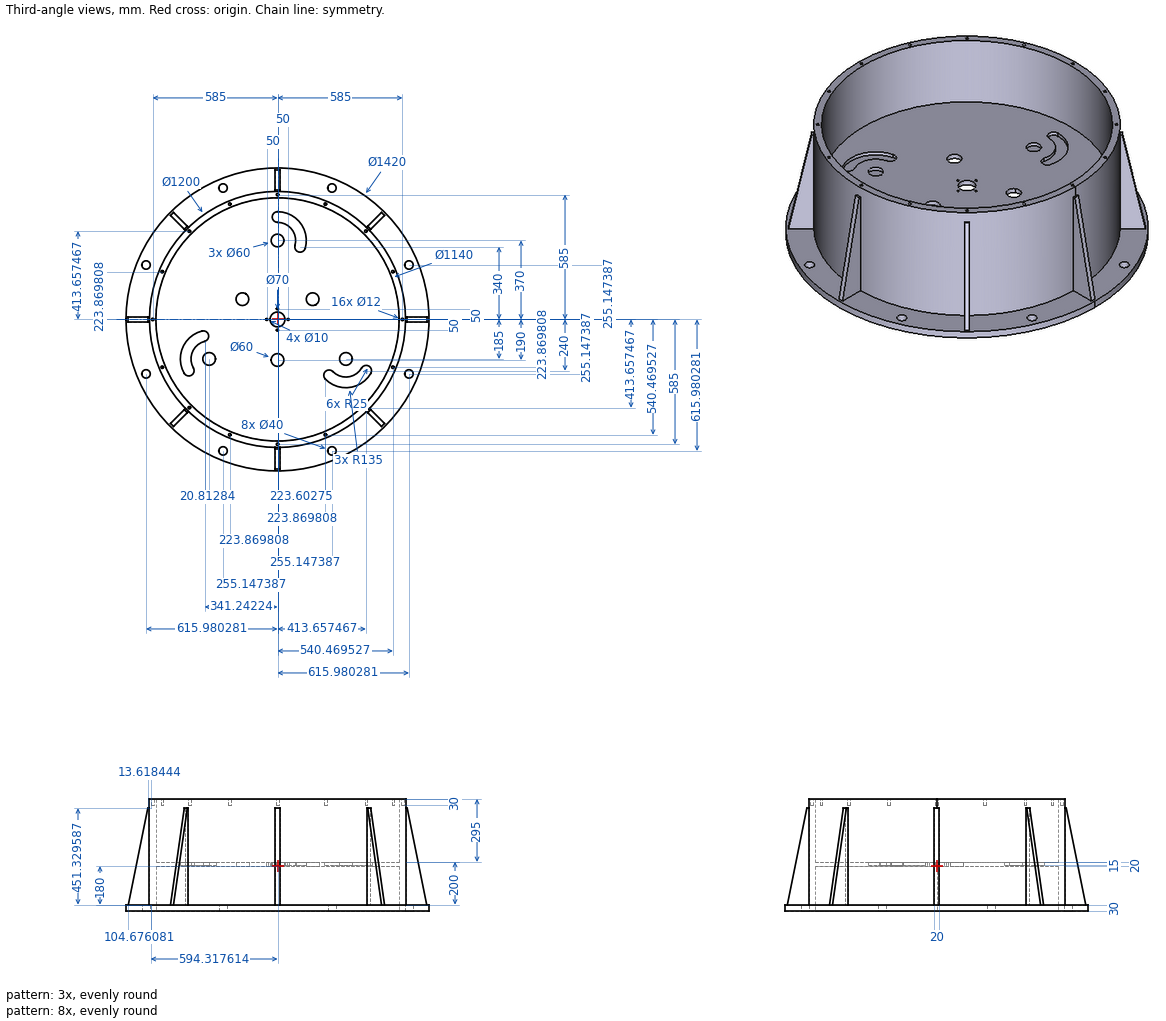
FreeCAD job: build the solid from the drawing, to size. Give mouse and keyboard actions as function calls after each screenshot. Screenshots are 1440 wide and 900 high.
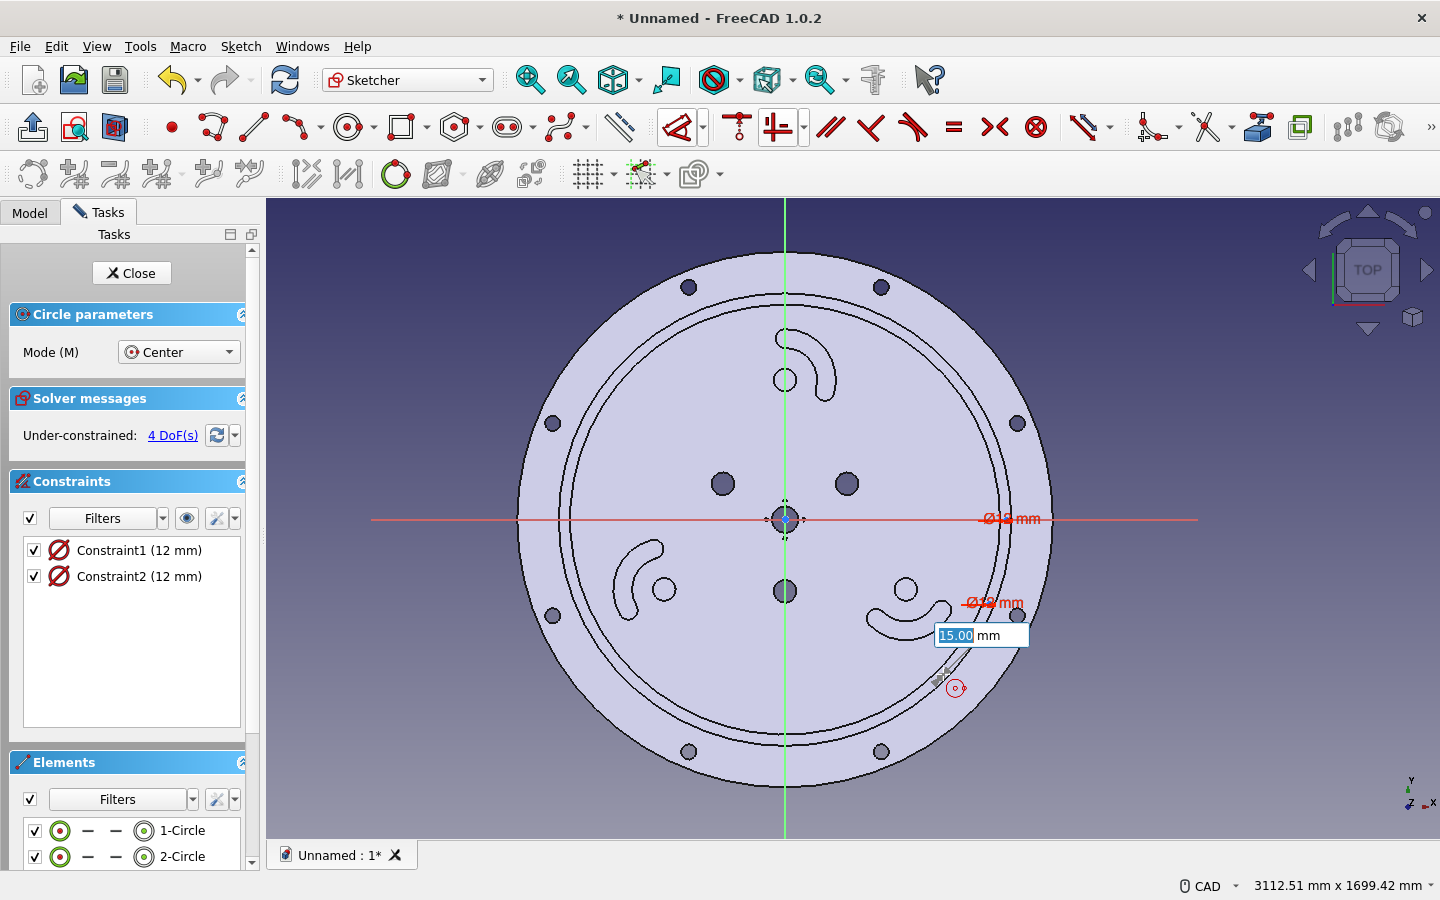
text(12)
key(Return)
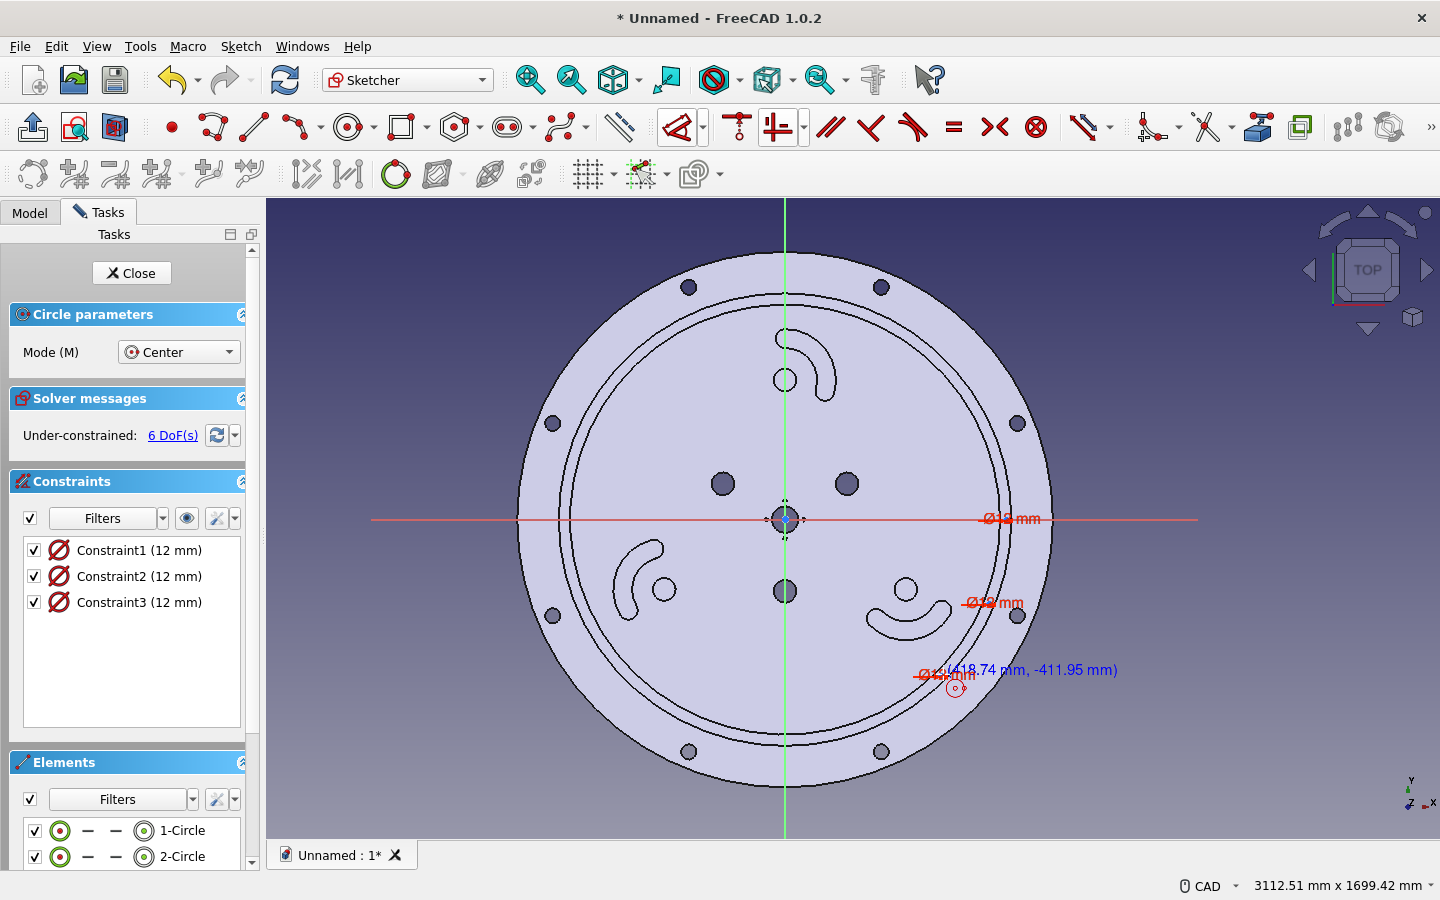
scroll(869, 723, up, 12)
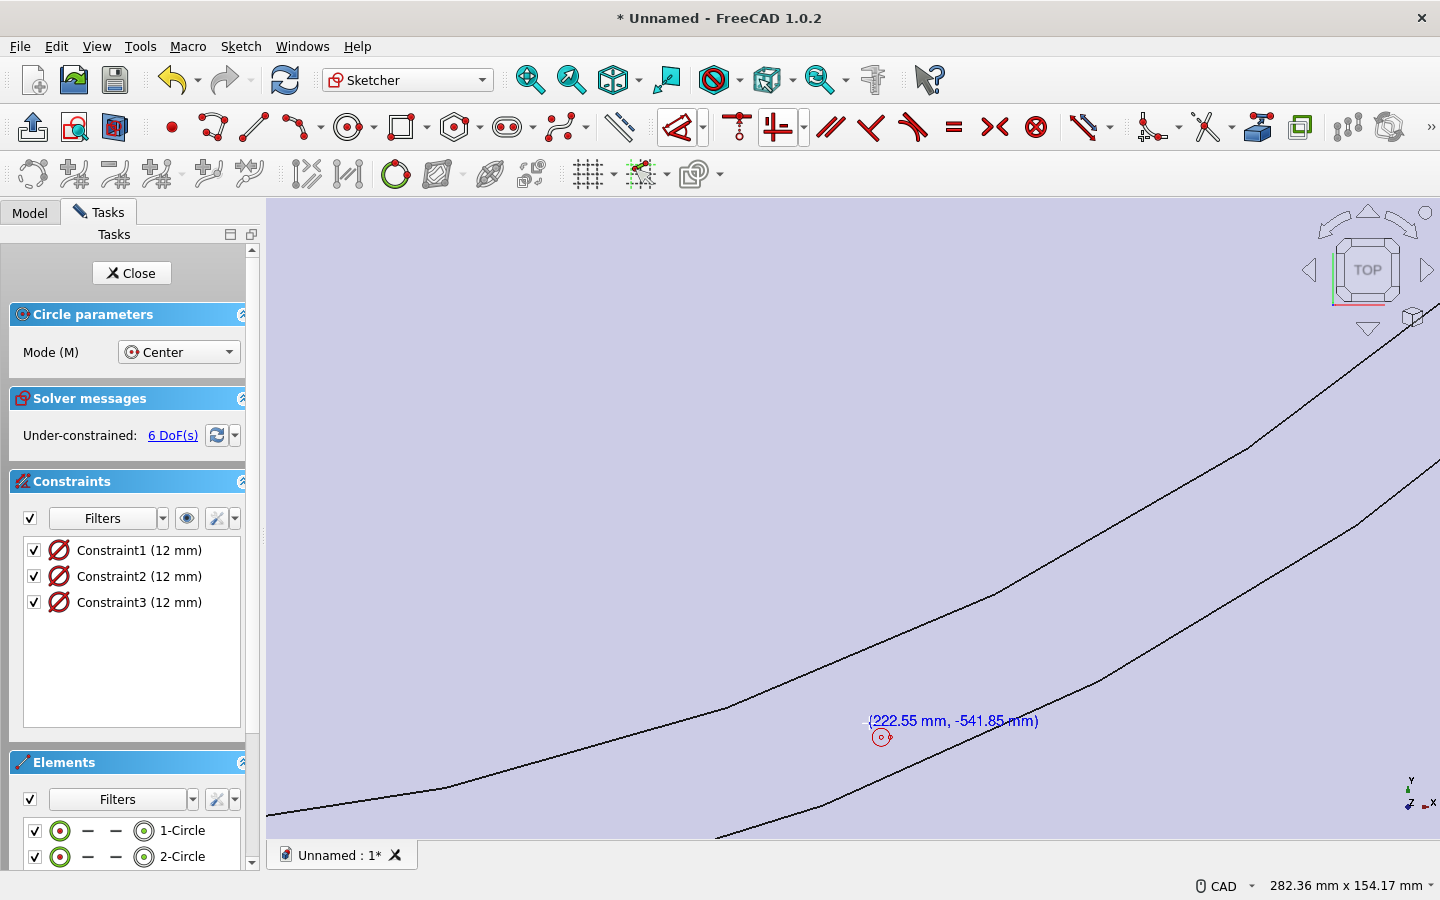
scroll(869, 723, down, 12)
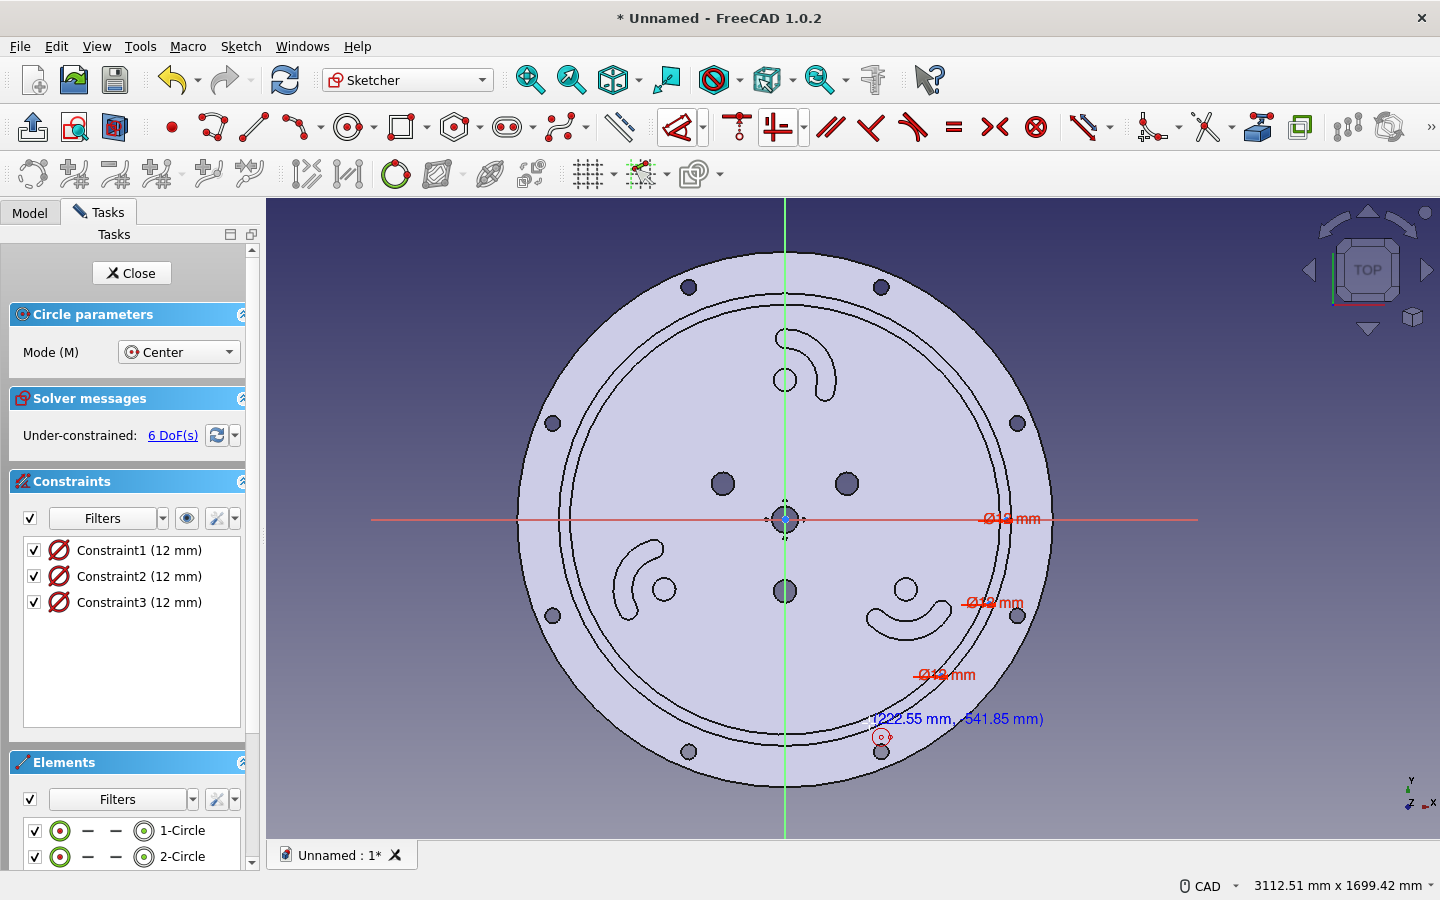
click(869, 723)
move(871, 722)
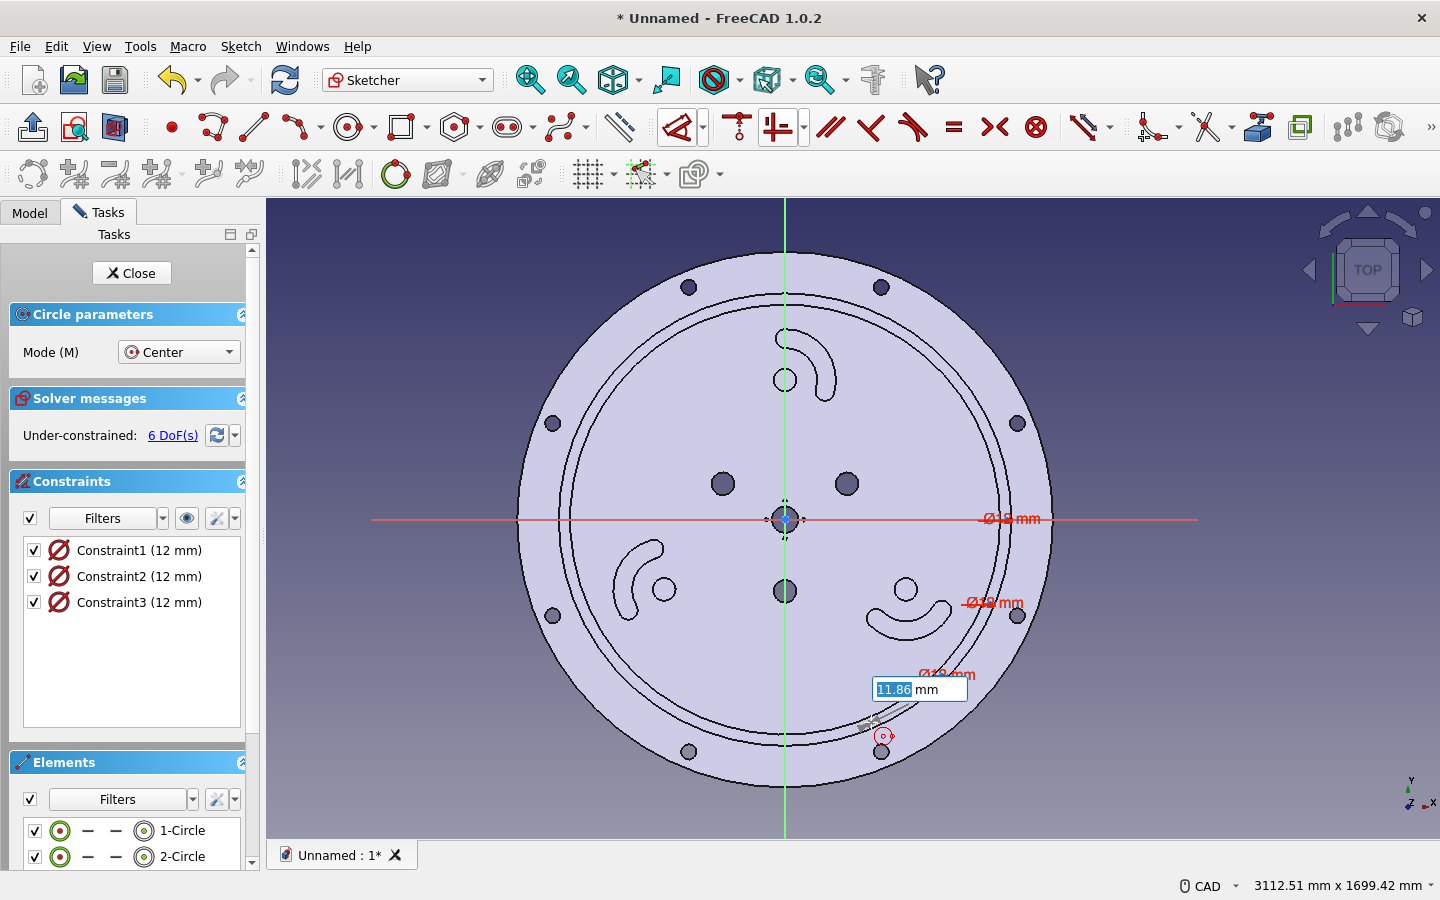
text(12)
key(Return)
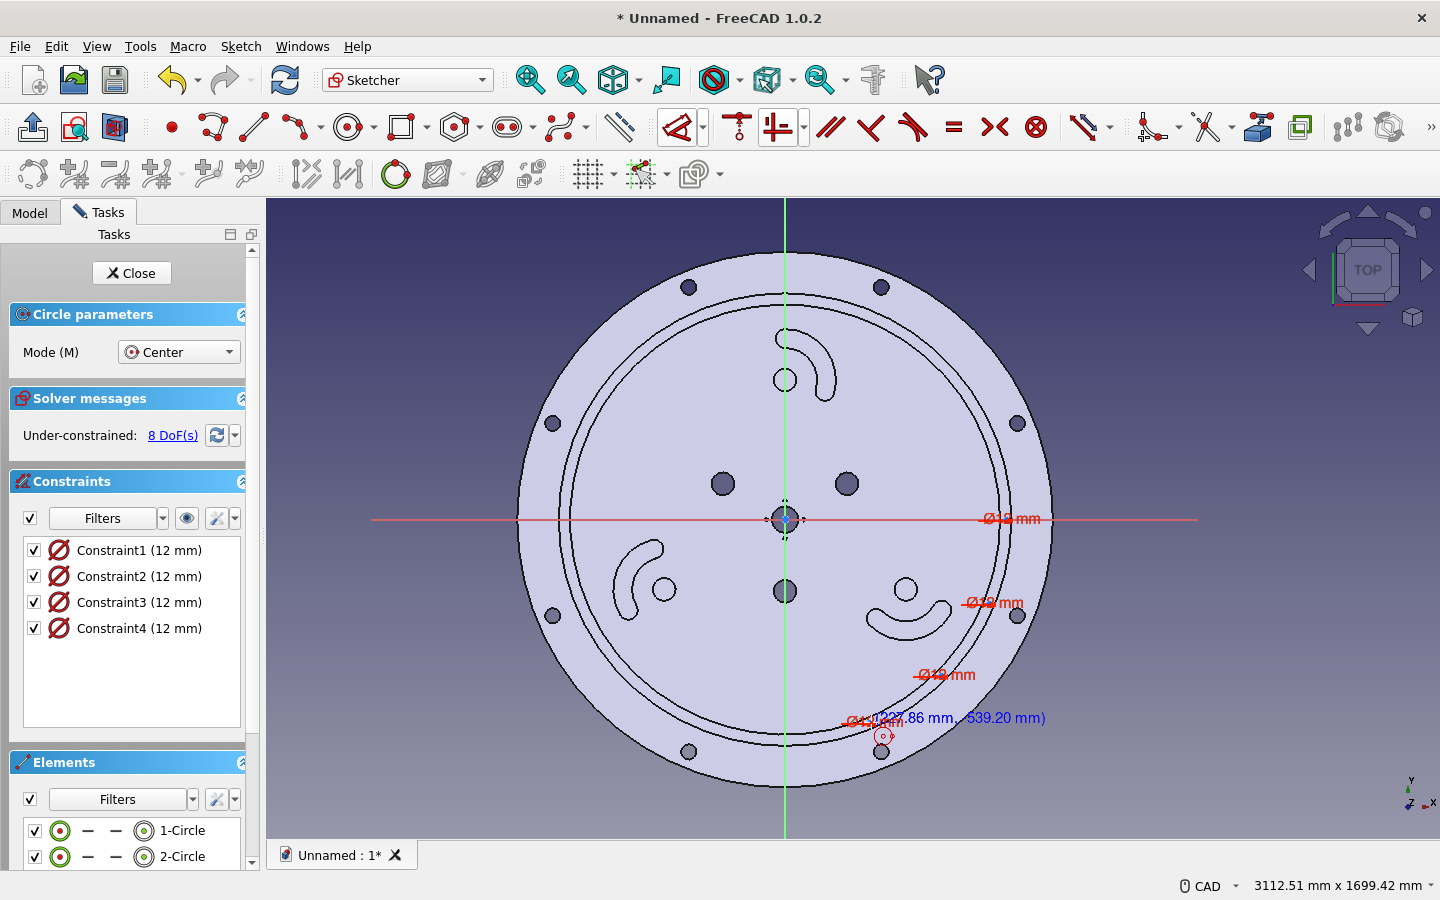
scroll(785, 740, up, 12)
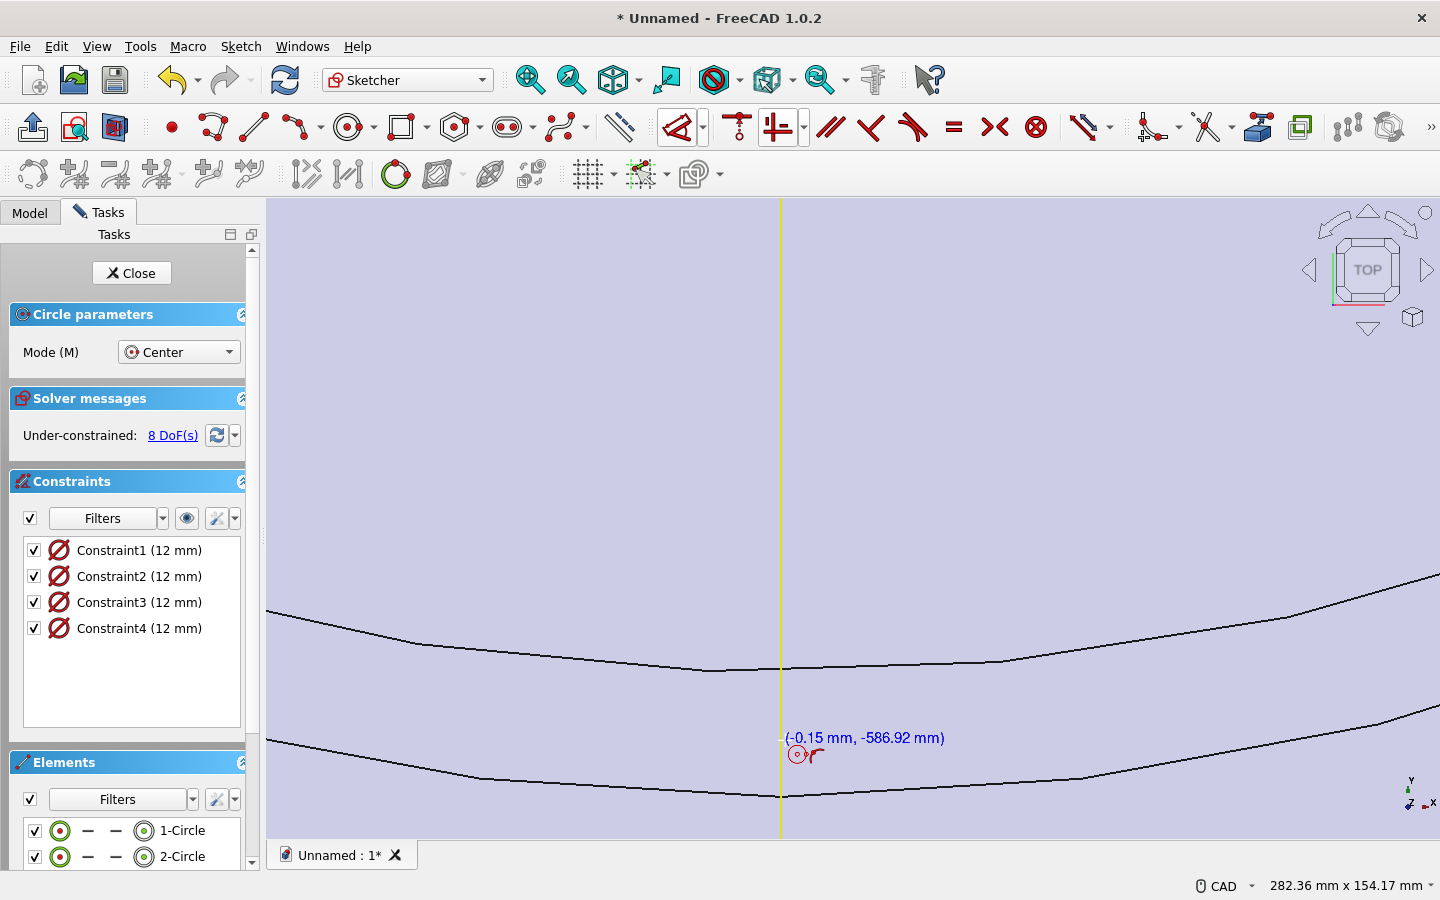
scroll(785, 740, down, 12)